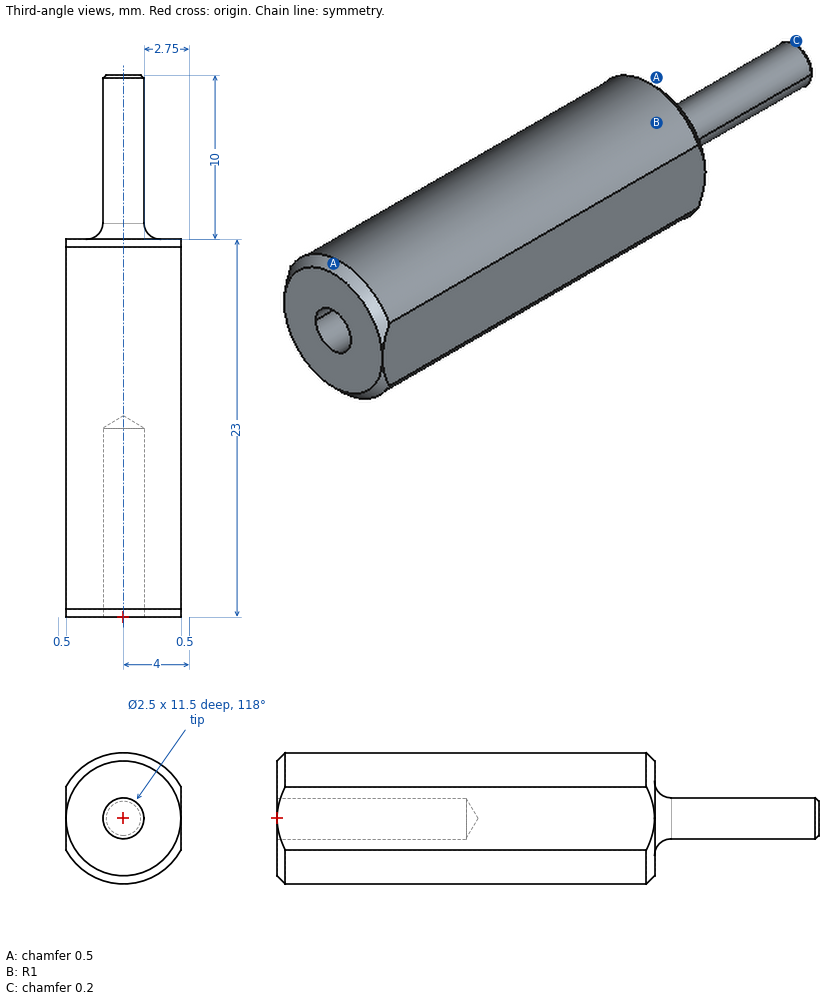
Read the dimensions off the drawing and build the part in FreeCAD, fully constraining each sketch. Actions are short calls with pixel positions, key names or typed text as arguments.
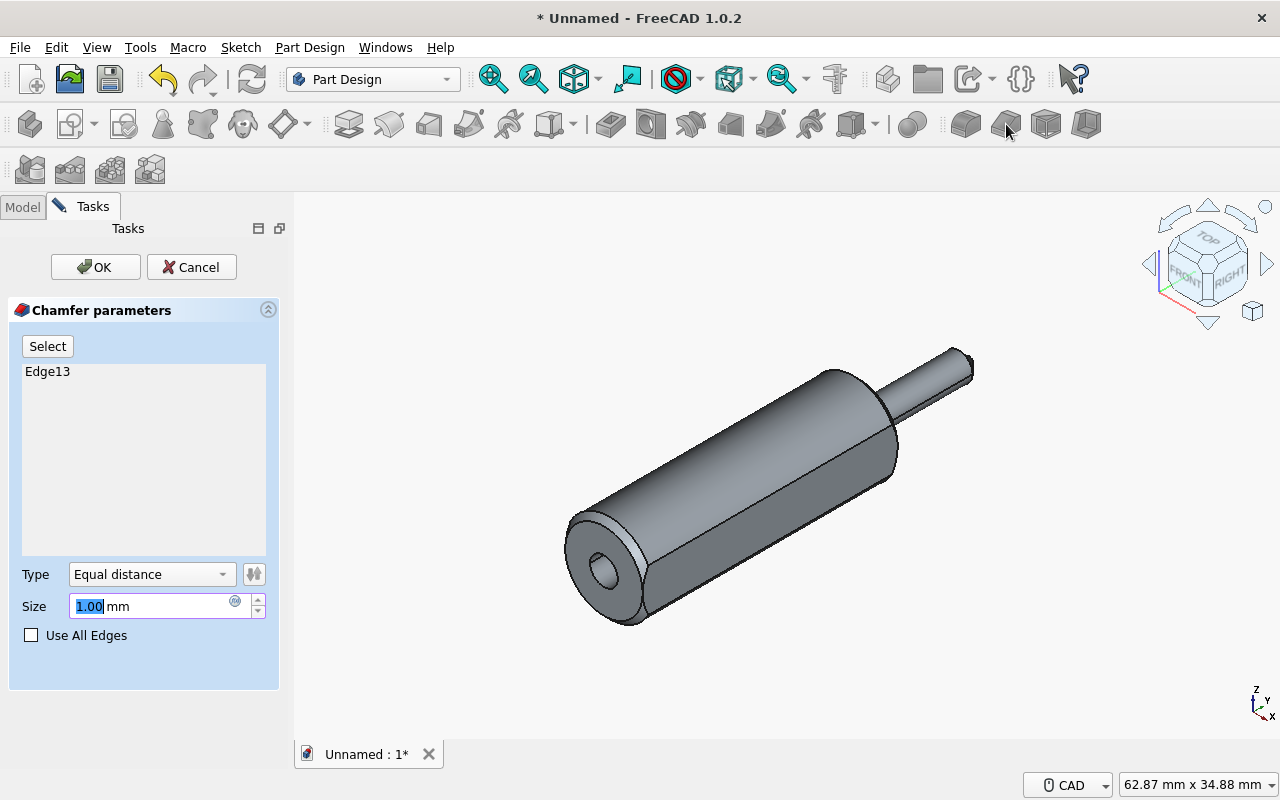
text(0.2)
key(Tab)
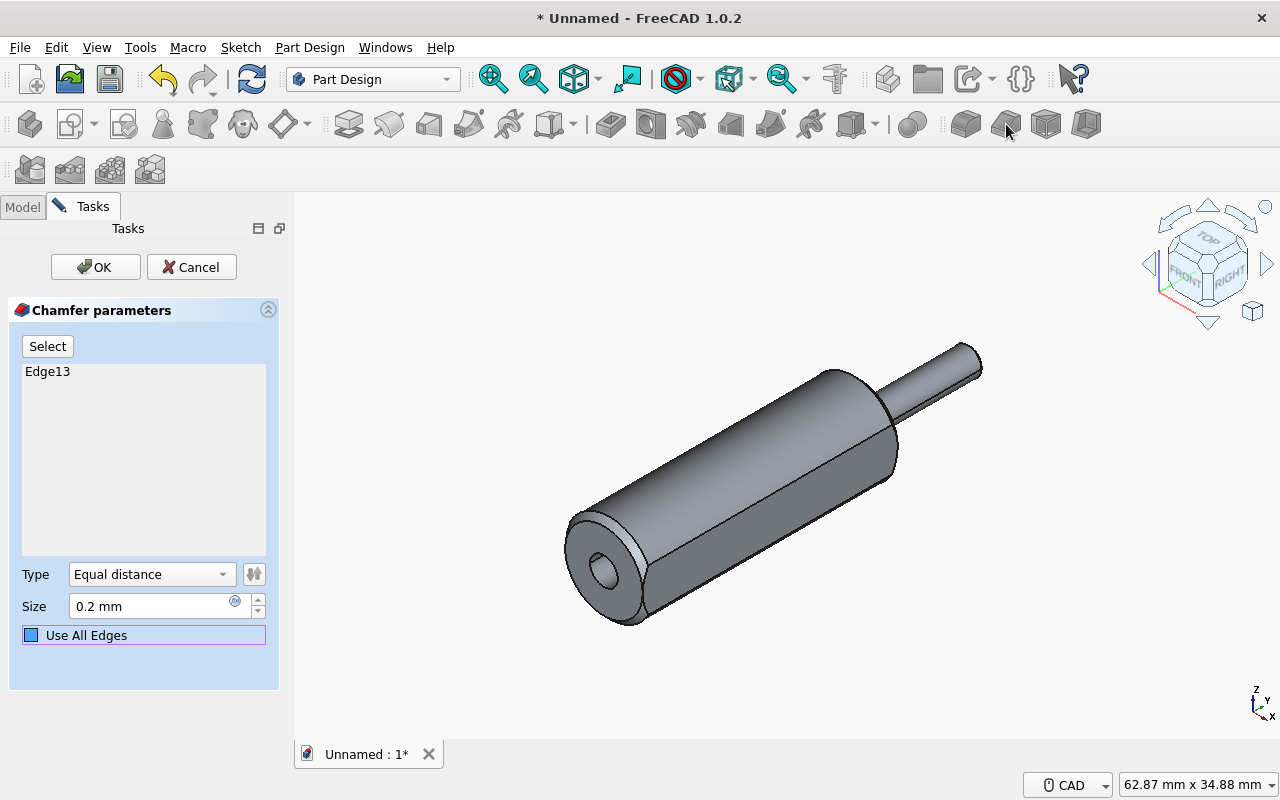
click(96, 267)